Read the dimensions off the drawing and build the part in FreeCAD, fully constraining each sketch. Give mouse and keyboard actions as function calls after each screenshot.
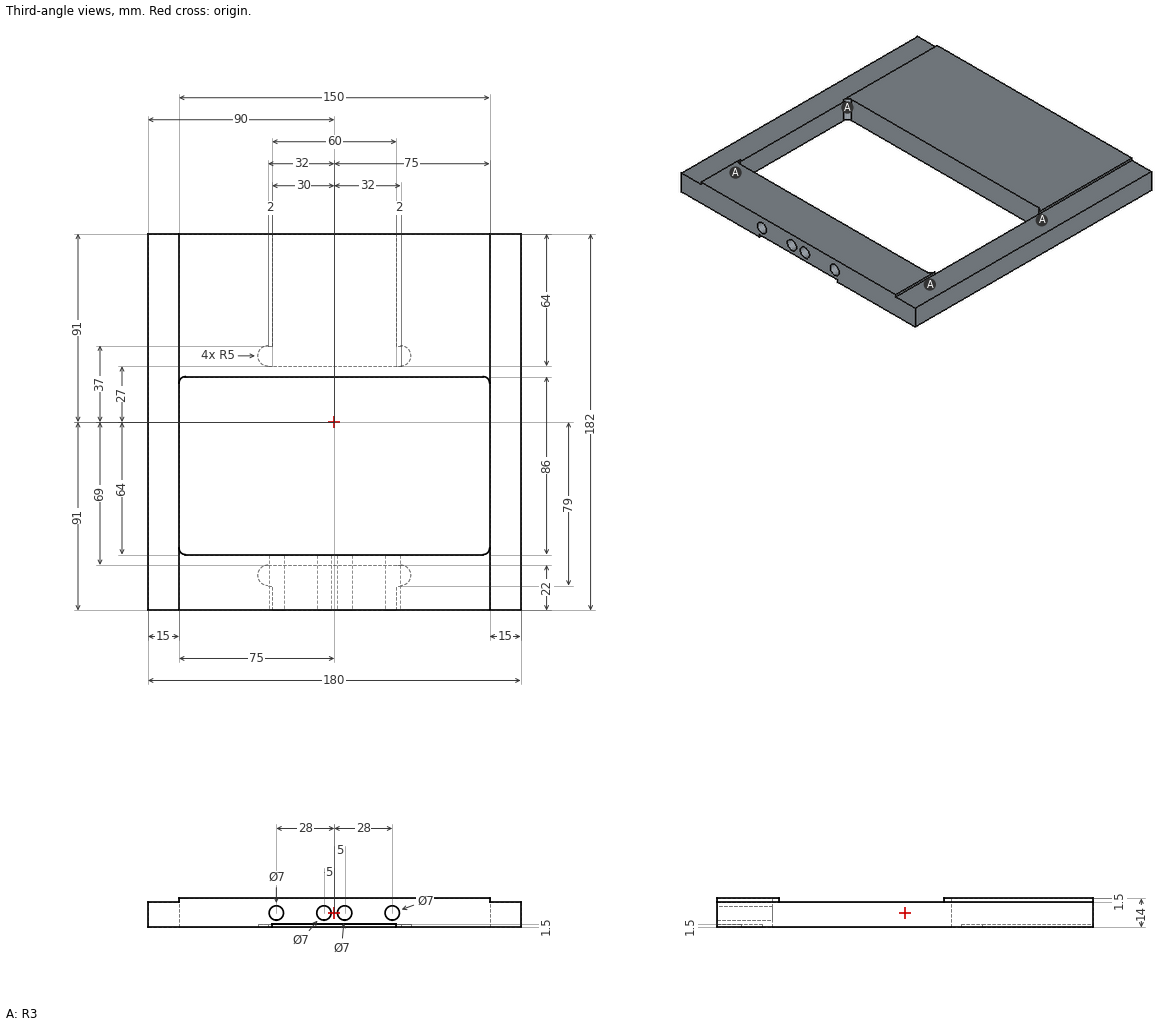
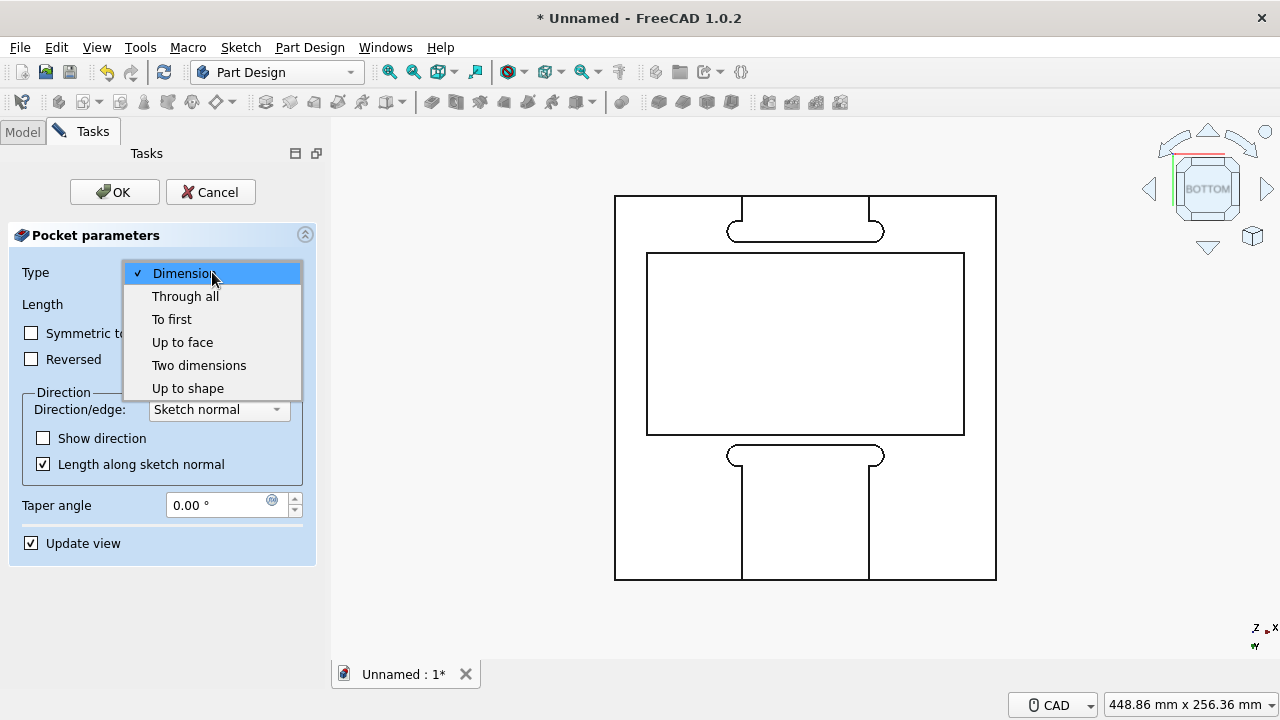
click(212, 320)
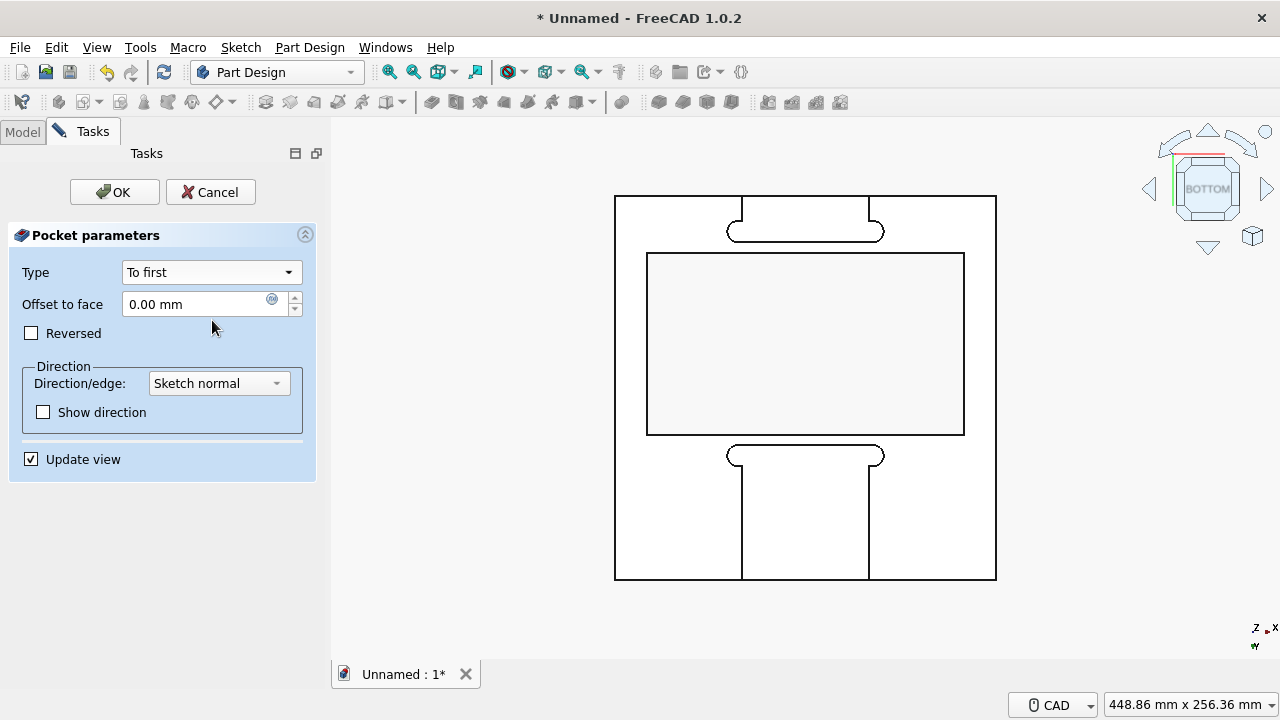
click(115, 192)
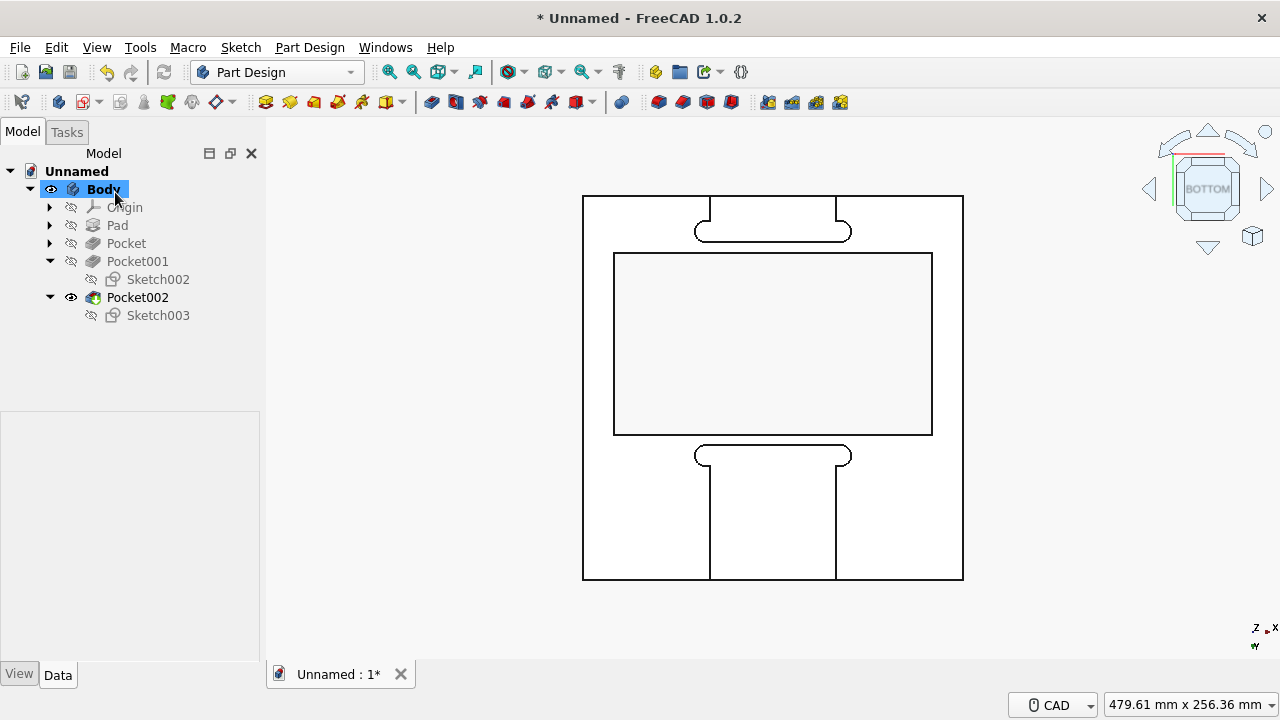
key(0)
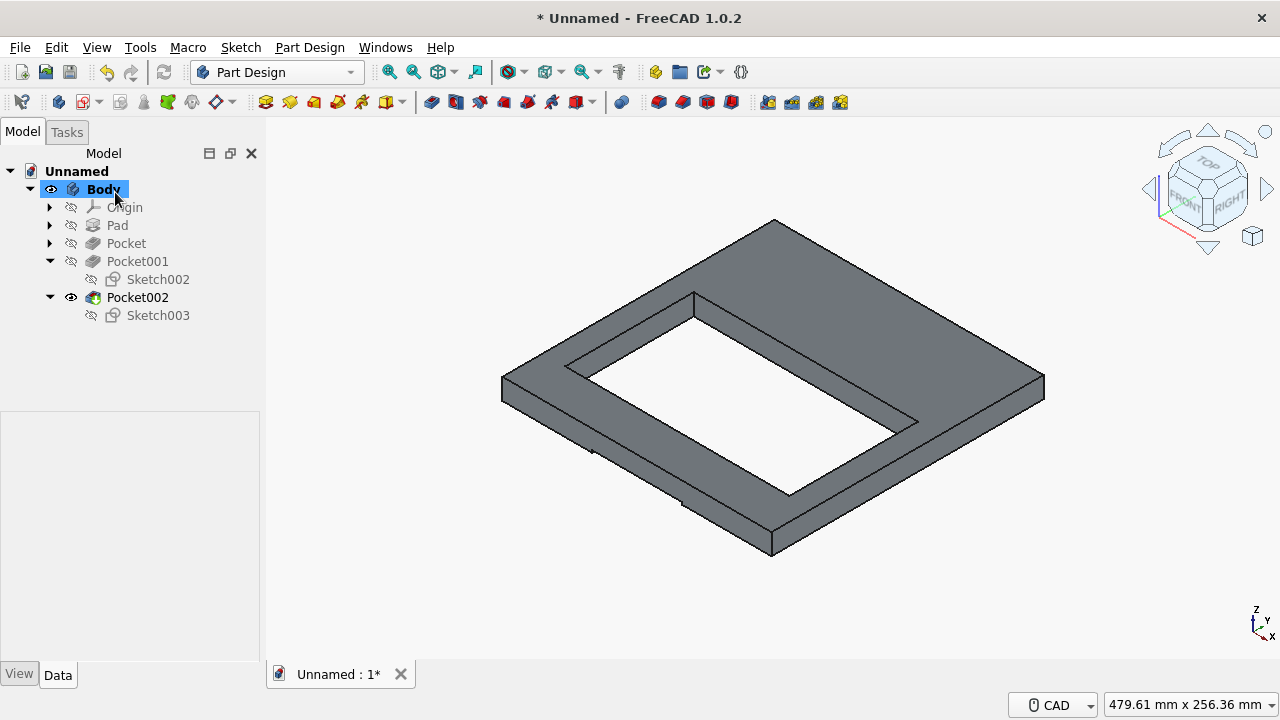
key(2)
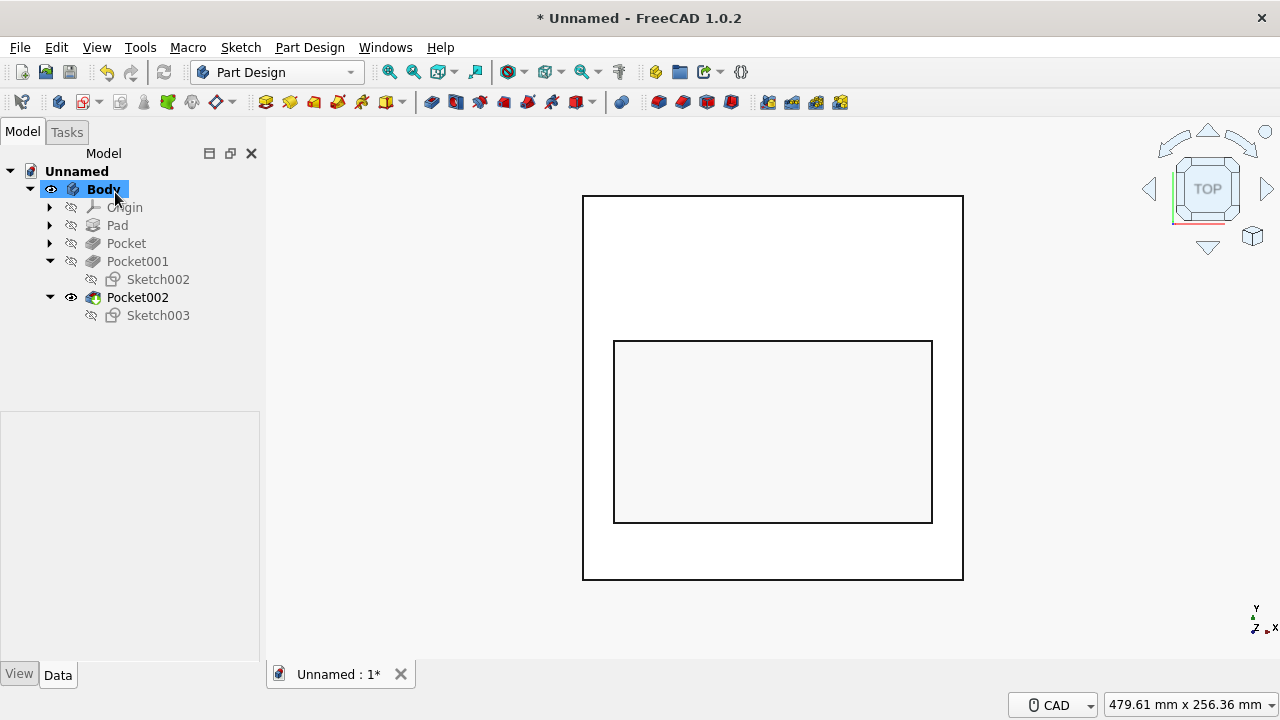
key(1)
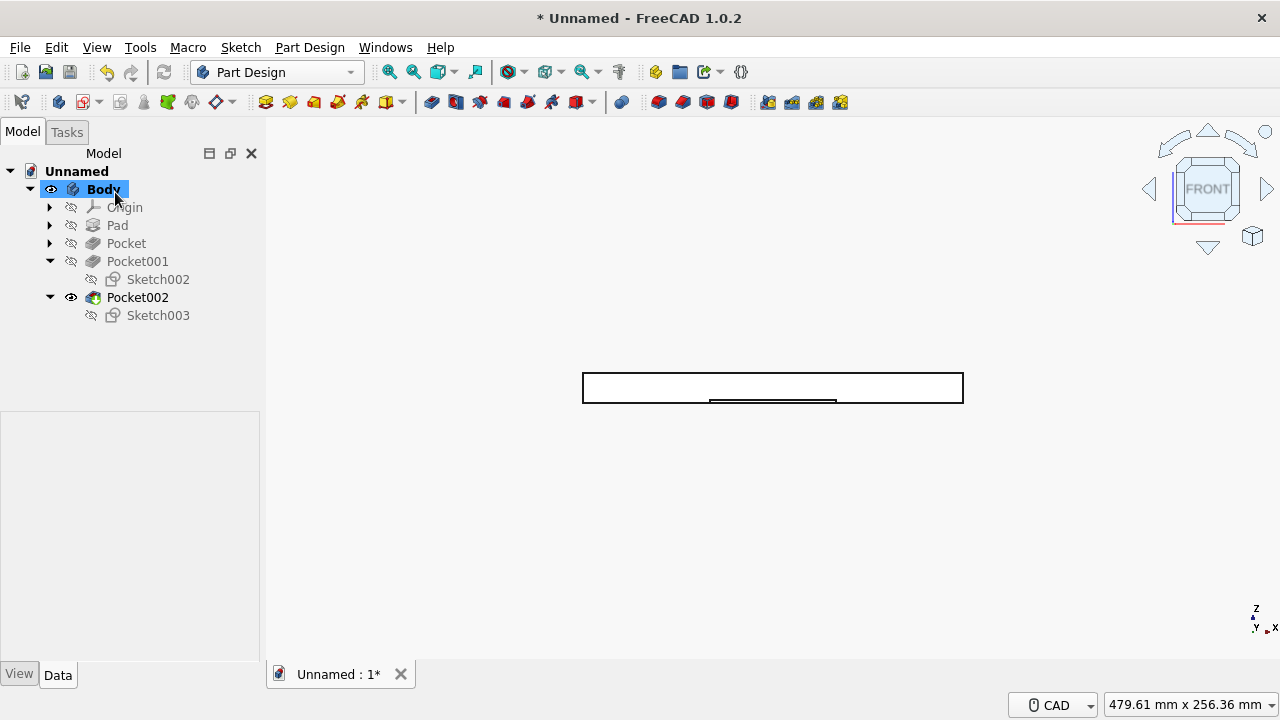
key(v)
key(f)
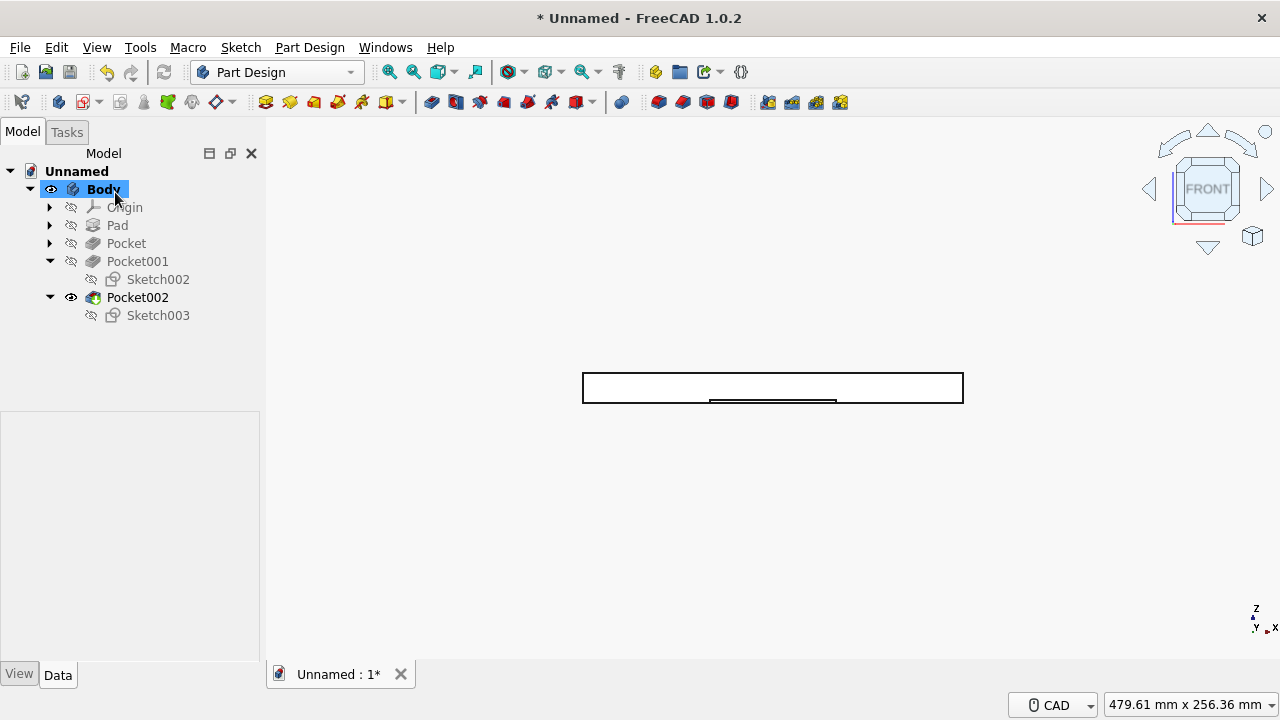
key(3)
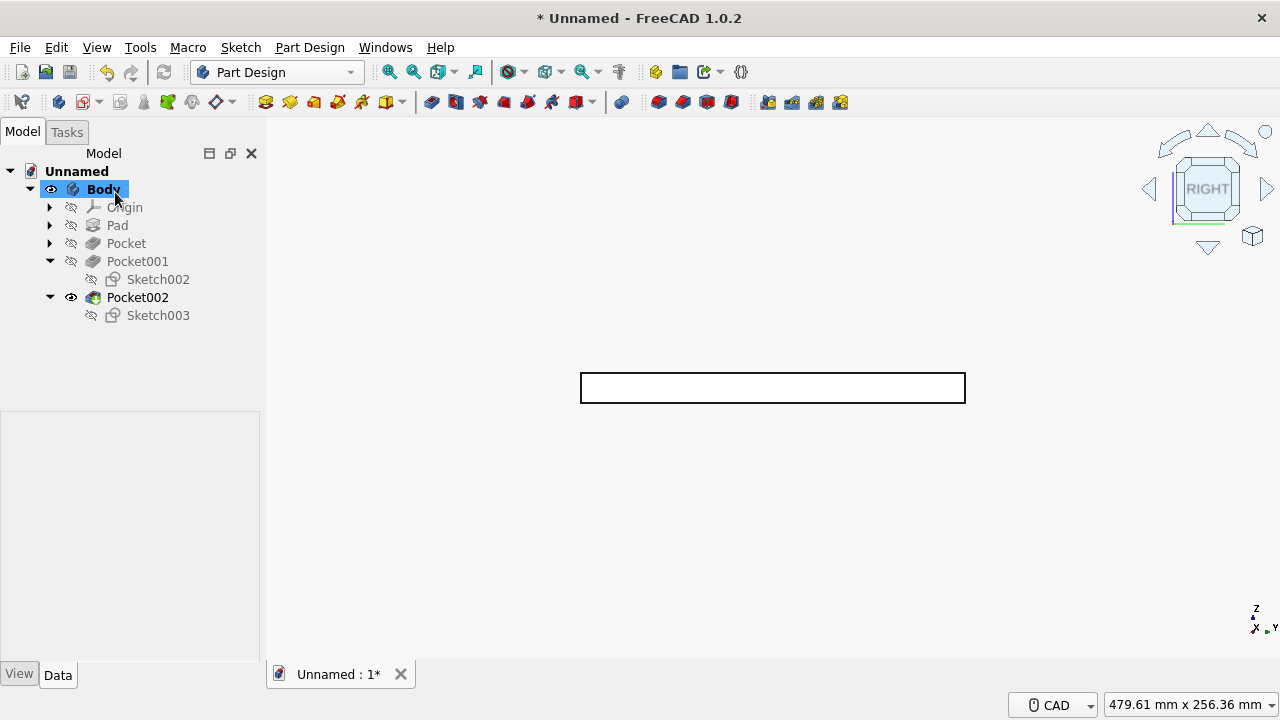
key(v)
key(f)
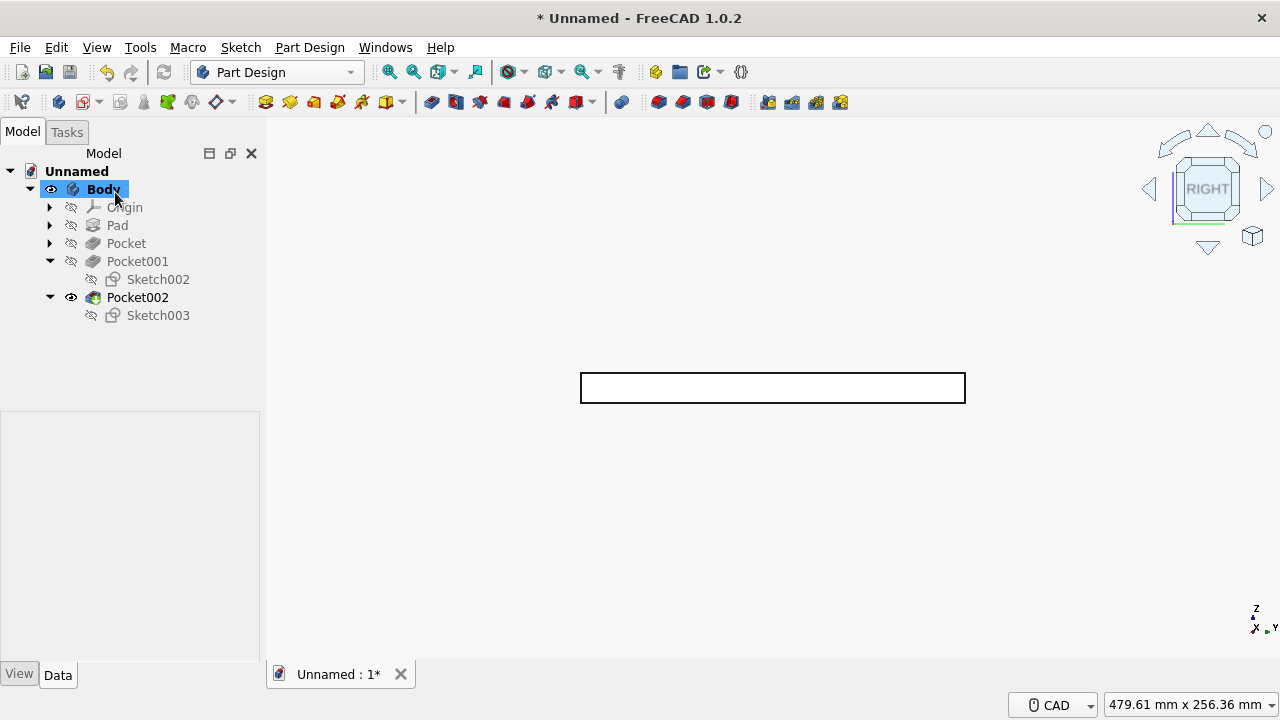
key(5)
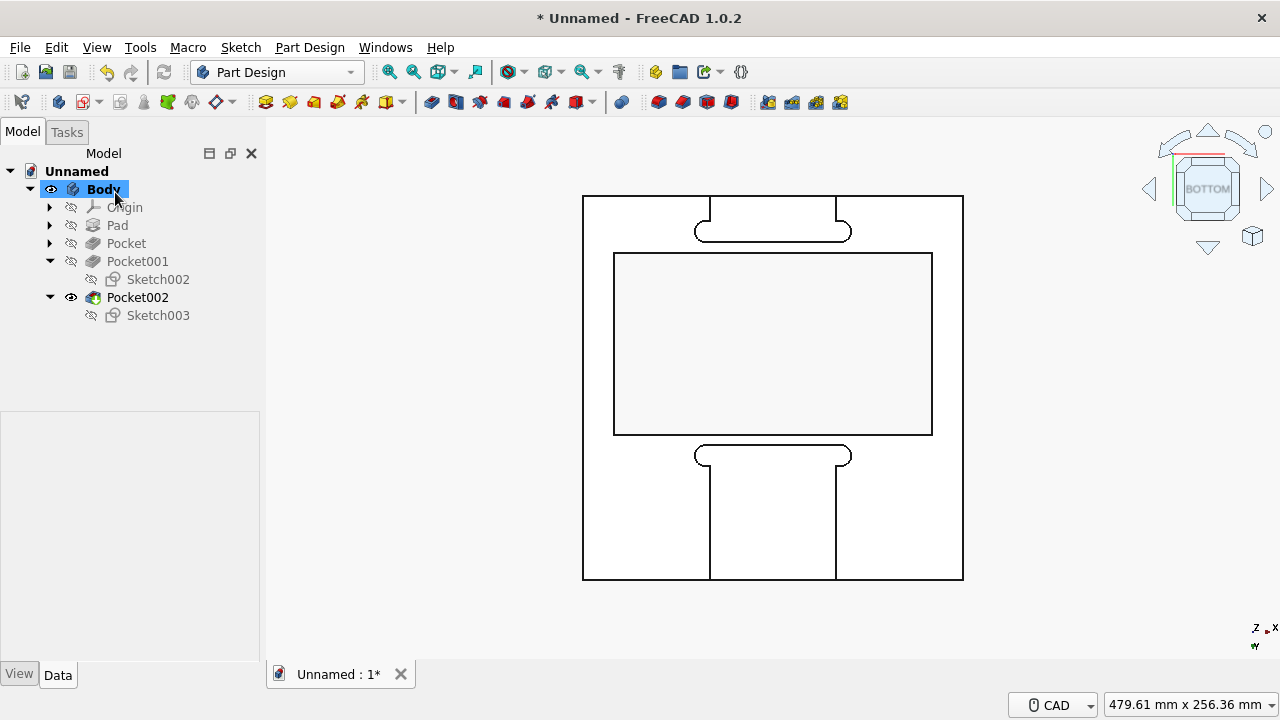
key(4)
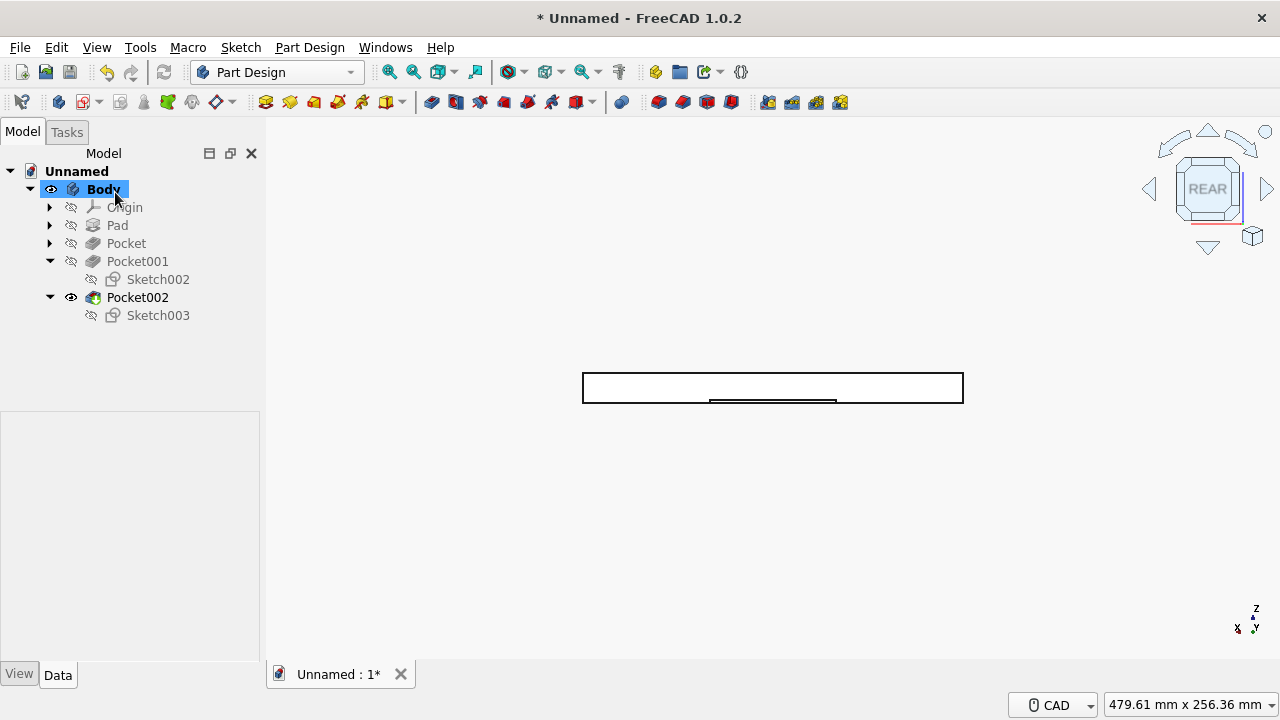
key(v)
key(f)